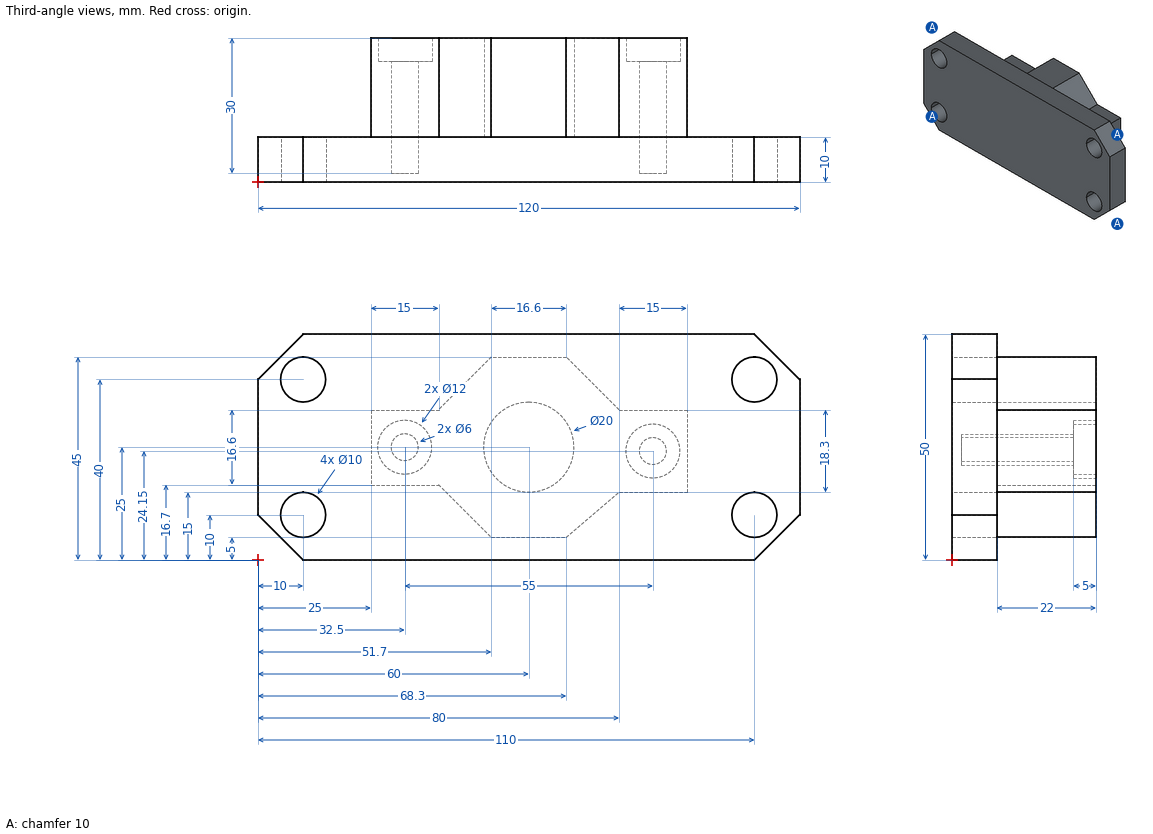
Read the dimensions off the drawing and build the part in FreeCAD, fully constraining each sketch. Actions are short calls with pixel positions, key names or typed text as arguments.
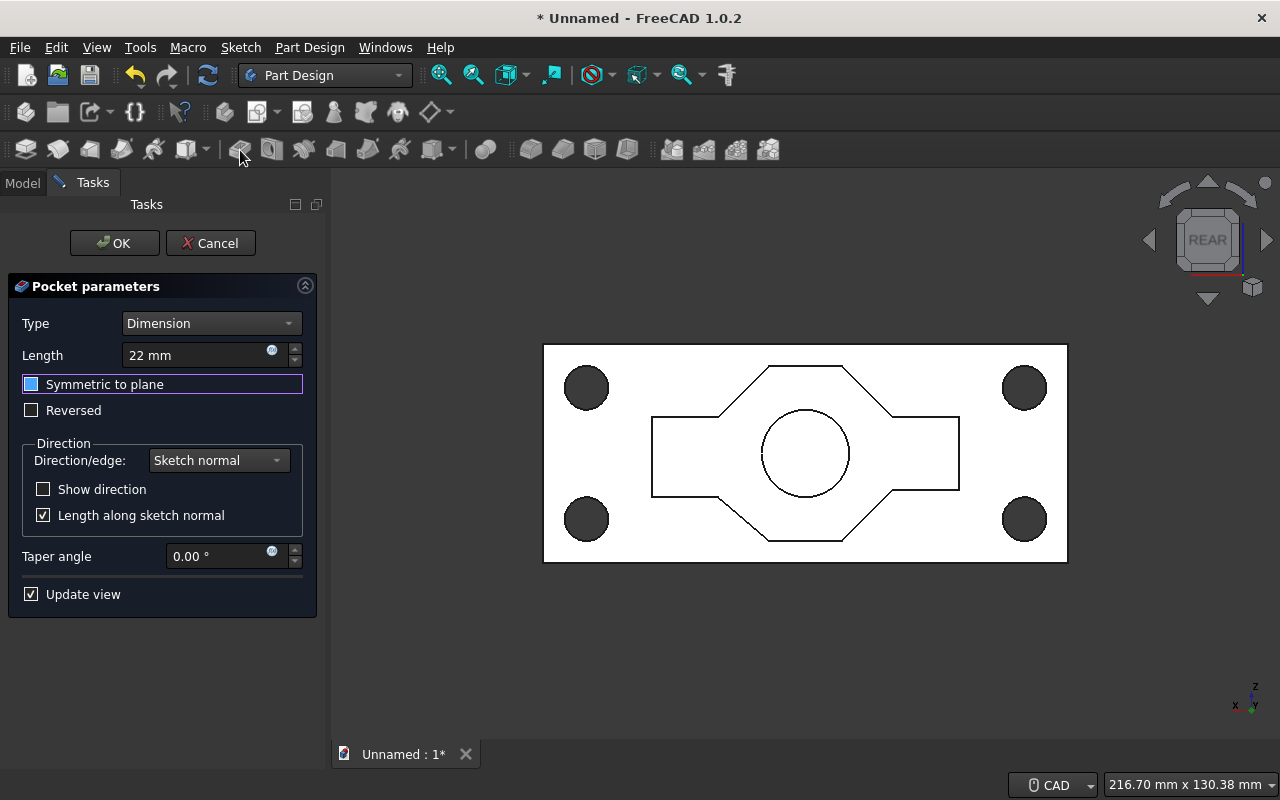
click(115, 243)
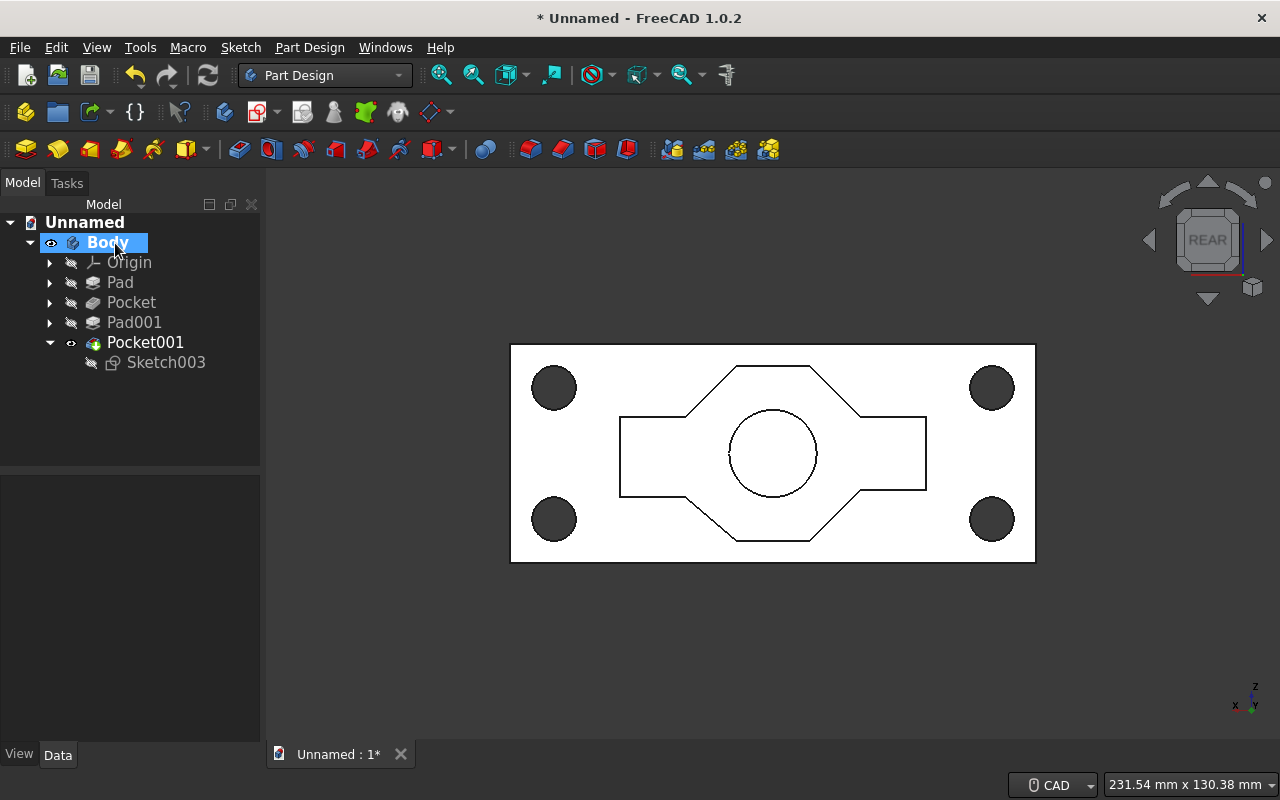
click(685, 452)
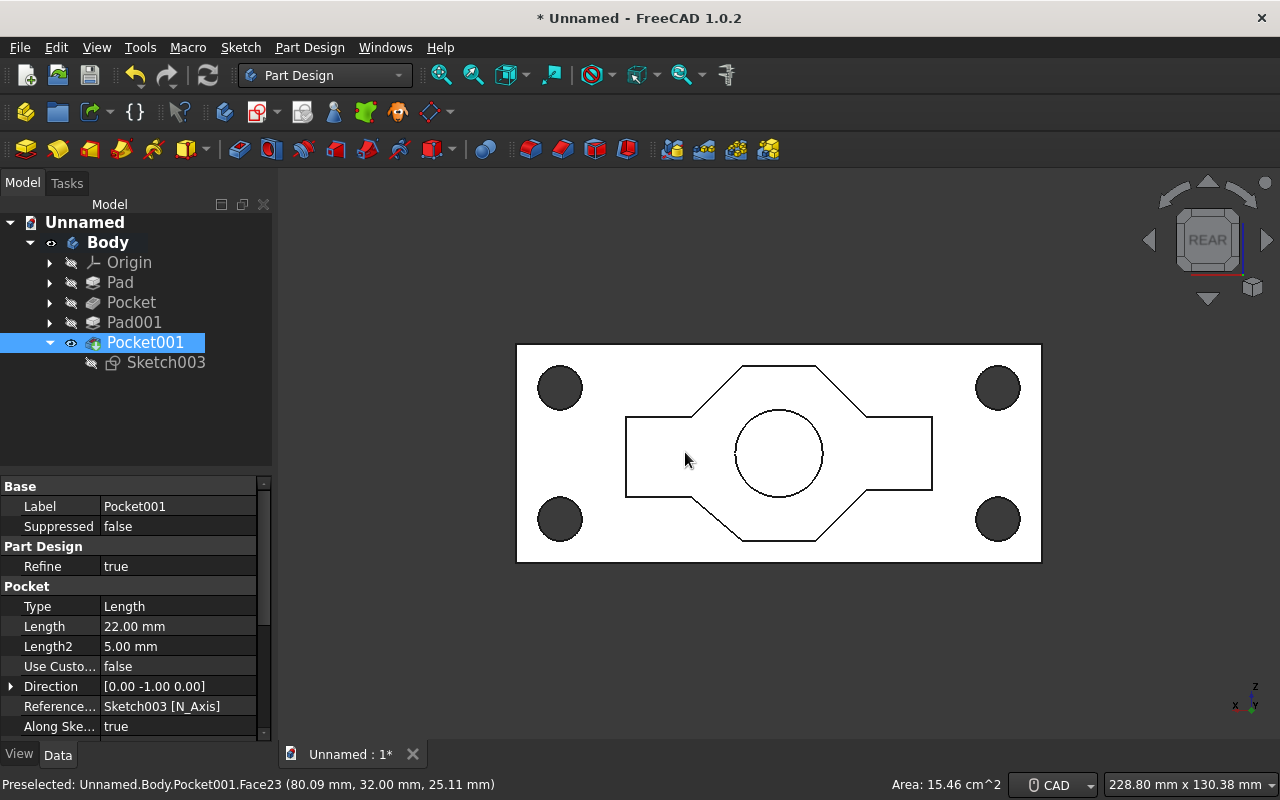
click(258, 112)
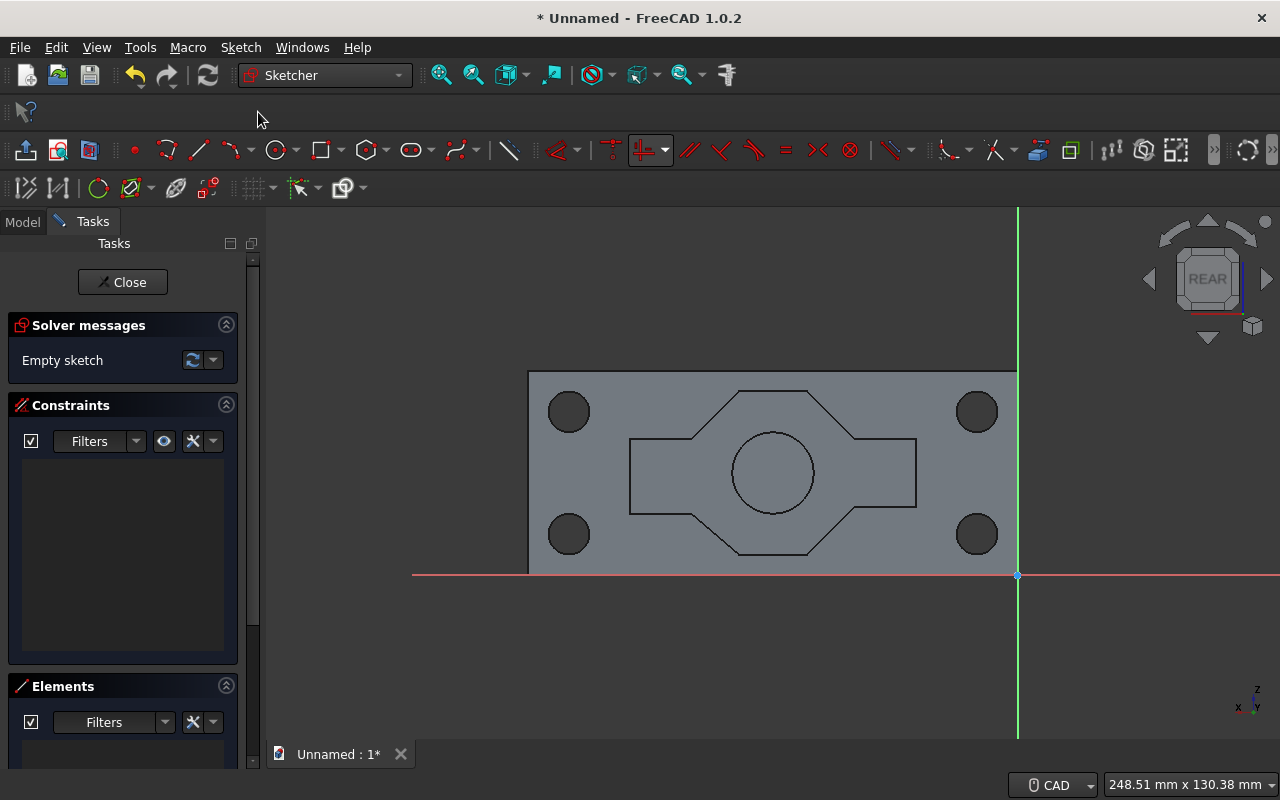
scroll(1095, 609, up, 2)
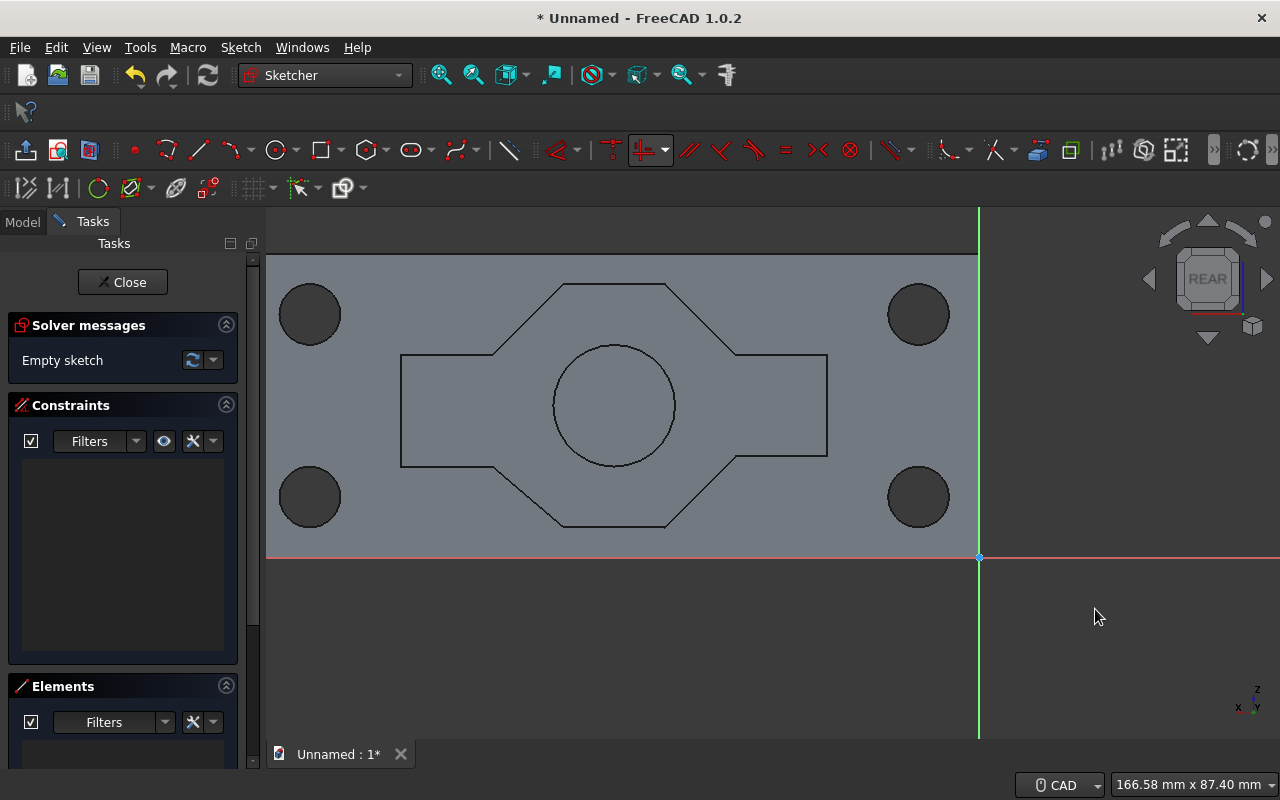
click(276, 150)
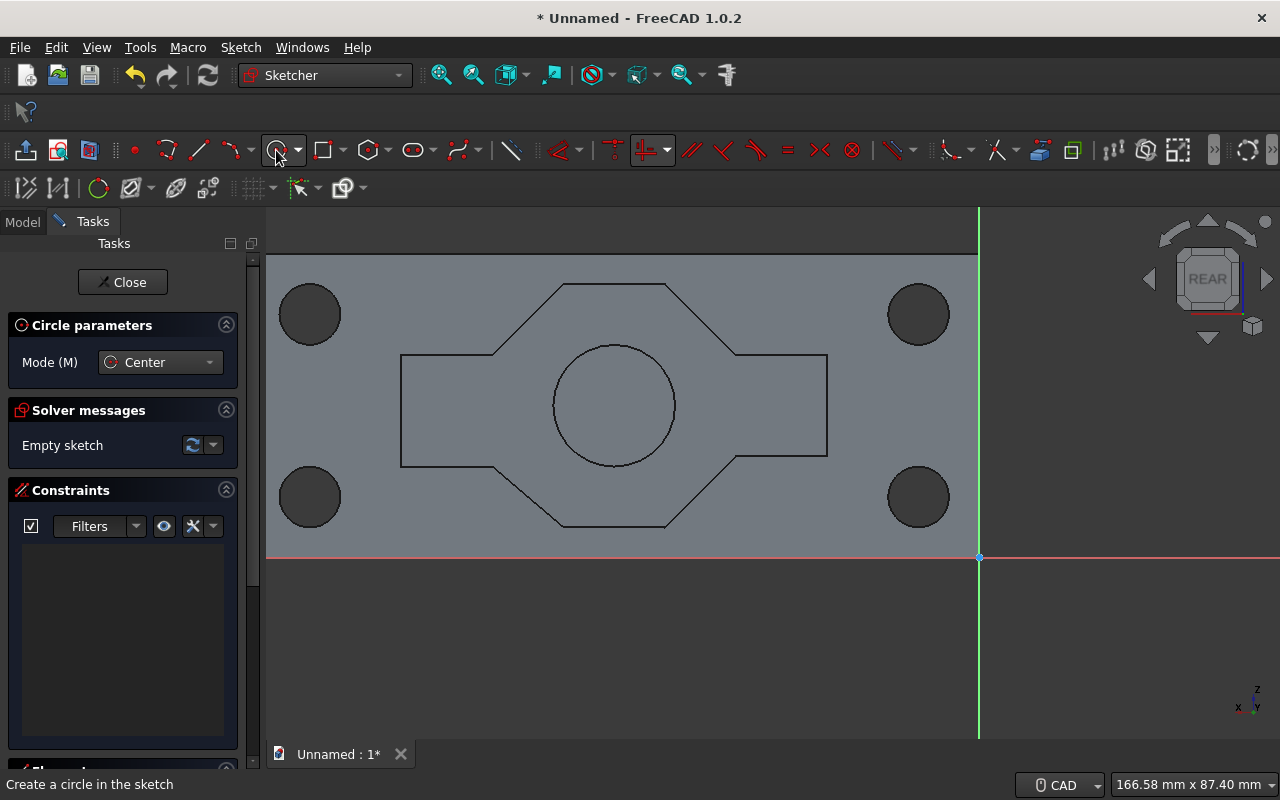
scroll(782, 406, up, 2)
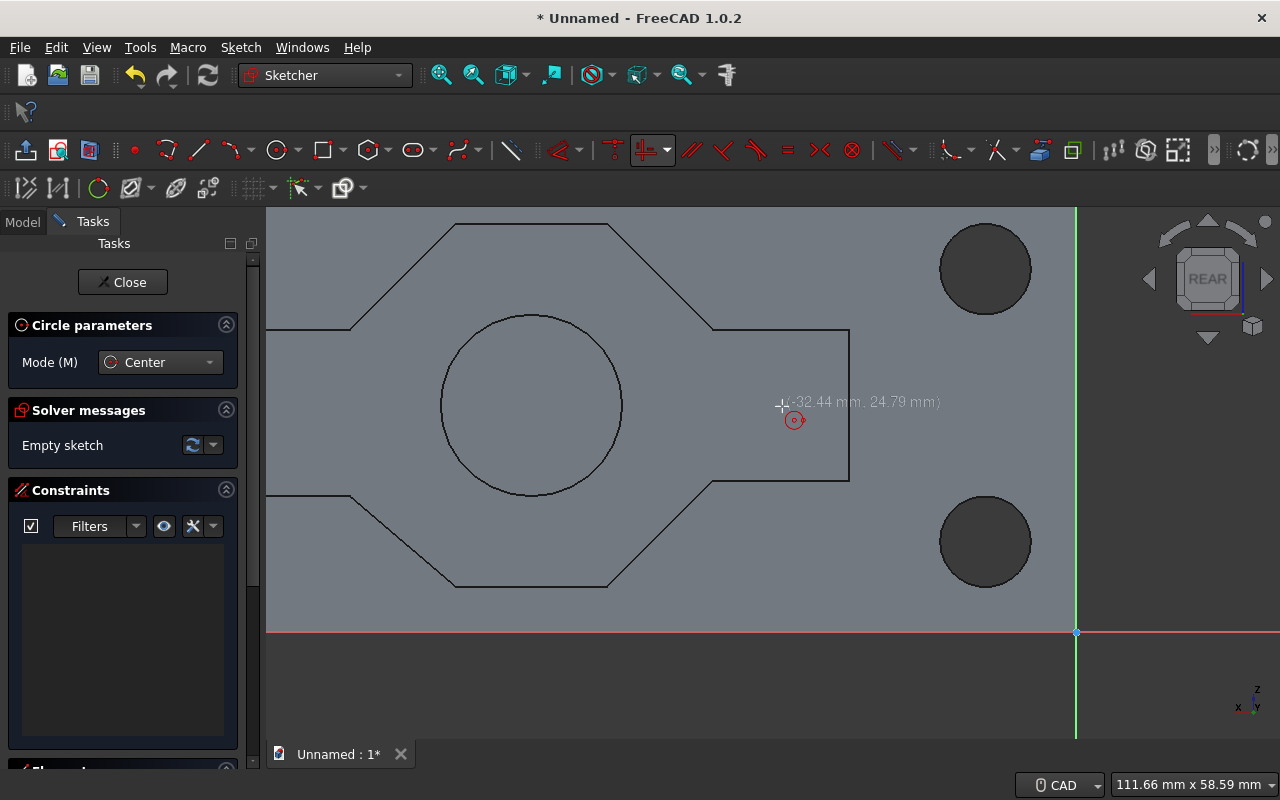
click(781, 405)
click(800, 386)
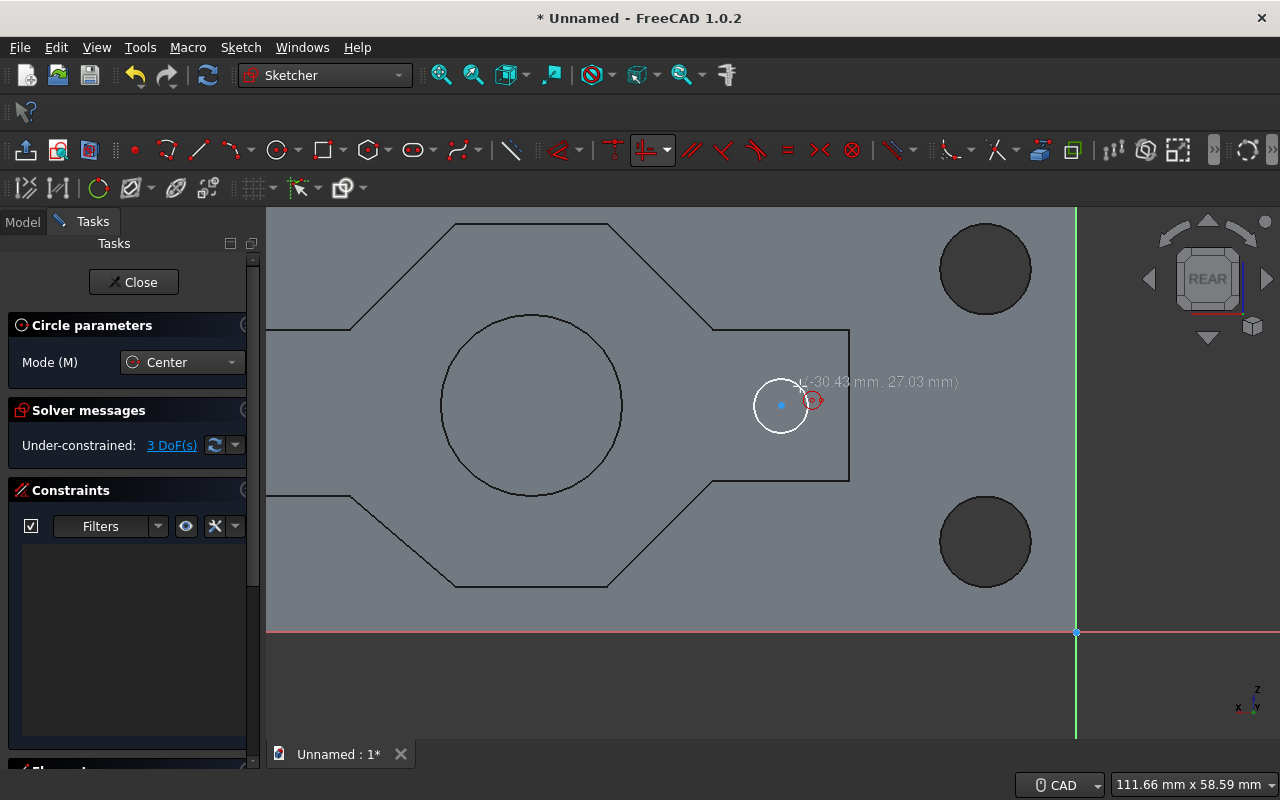
scroll(784, 407, down, 2)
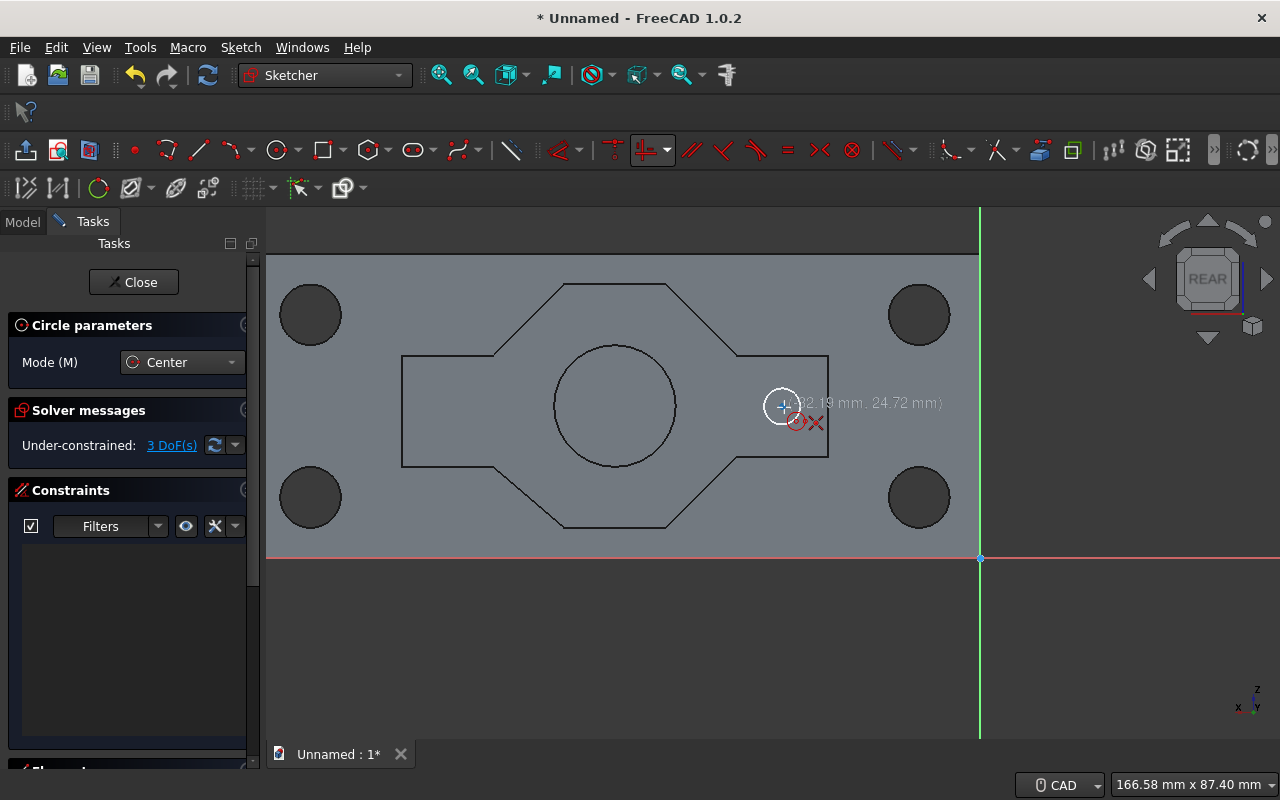
scroll(447, 411, up, 2)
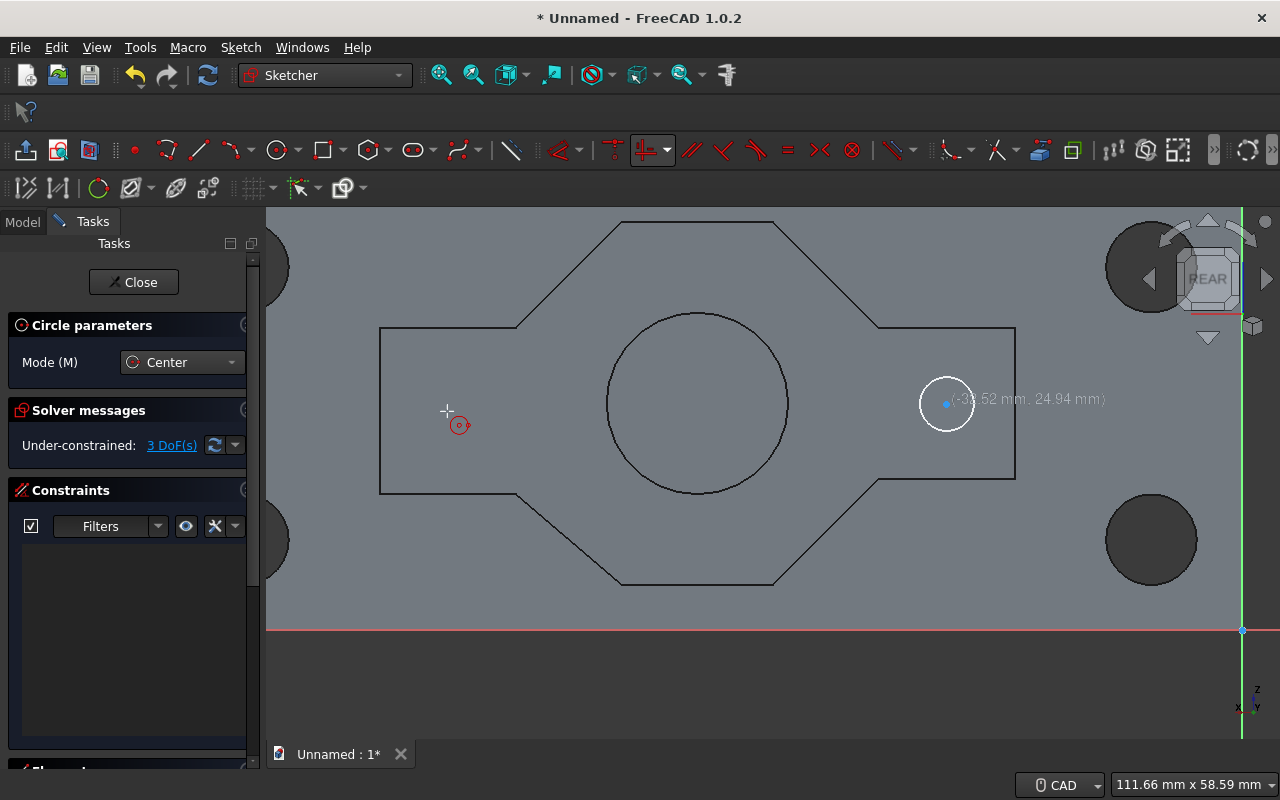
click(448, 411)
click(467, 392)
key(Escape)